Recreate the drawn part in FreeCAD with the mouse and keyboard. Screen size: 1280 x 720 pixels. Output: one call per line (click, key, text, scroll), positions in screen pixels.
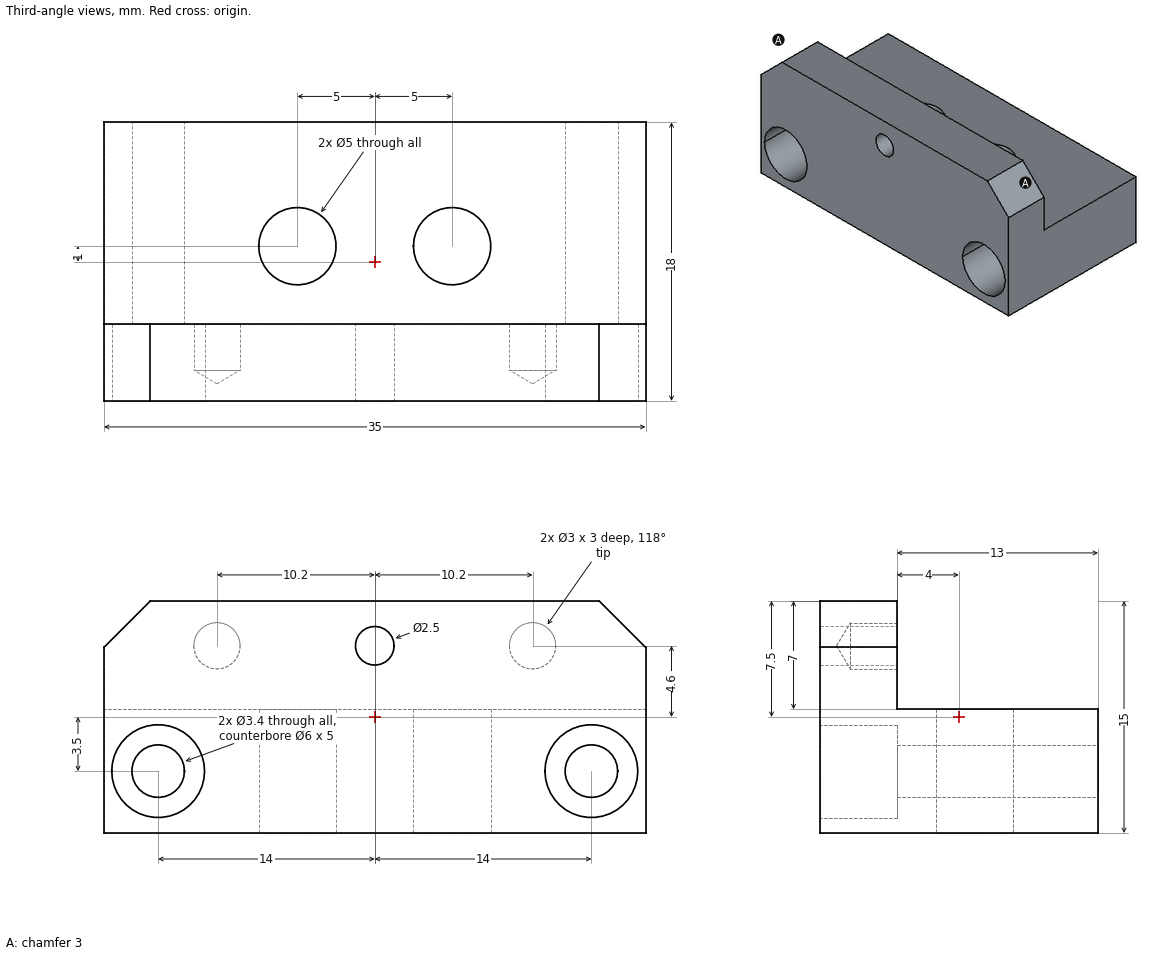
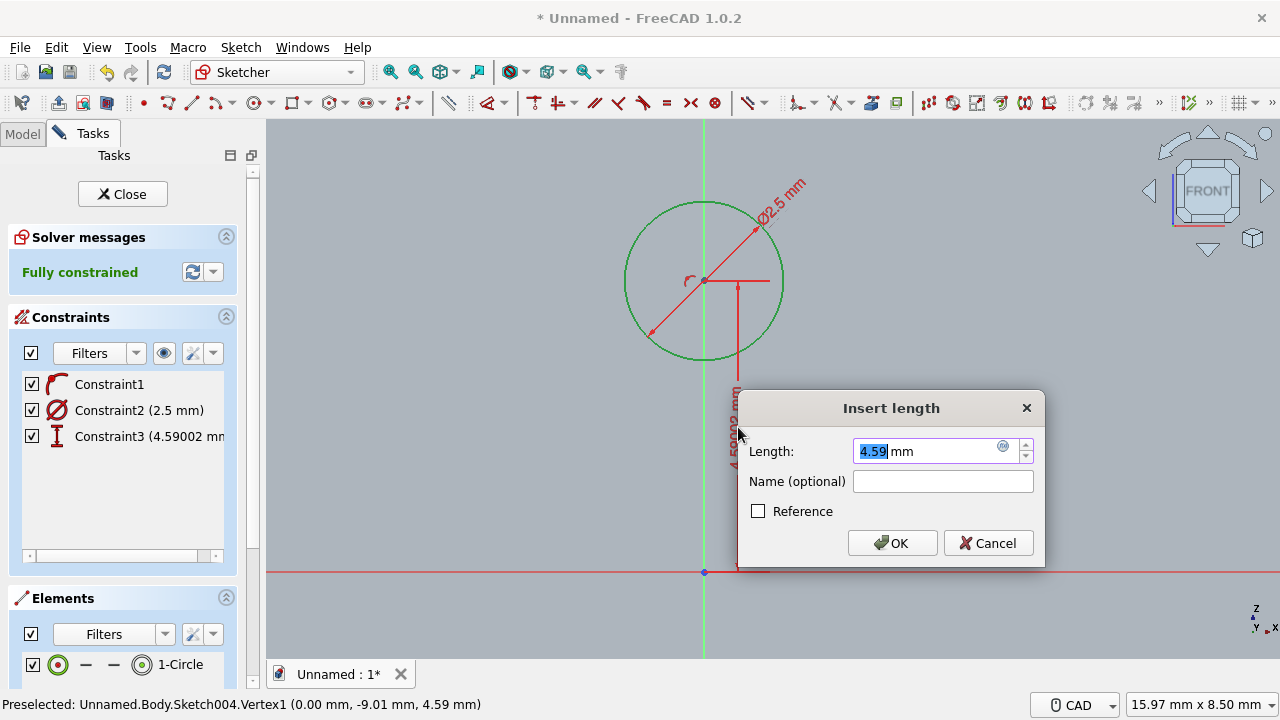
text(4.6)
key(Return)
key(Escape)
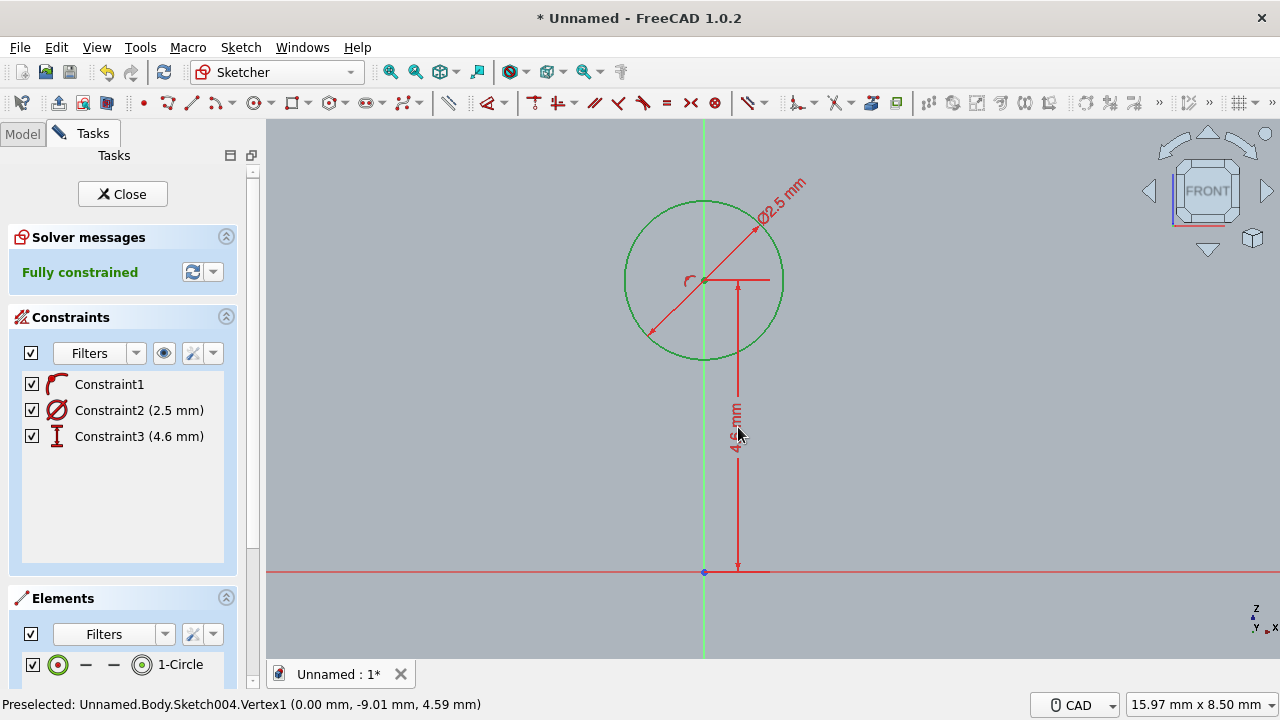
click(123, 194)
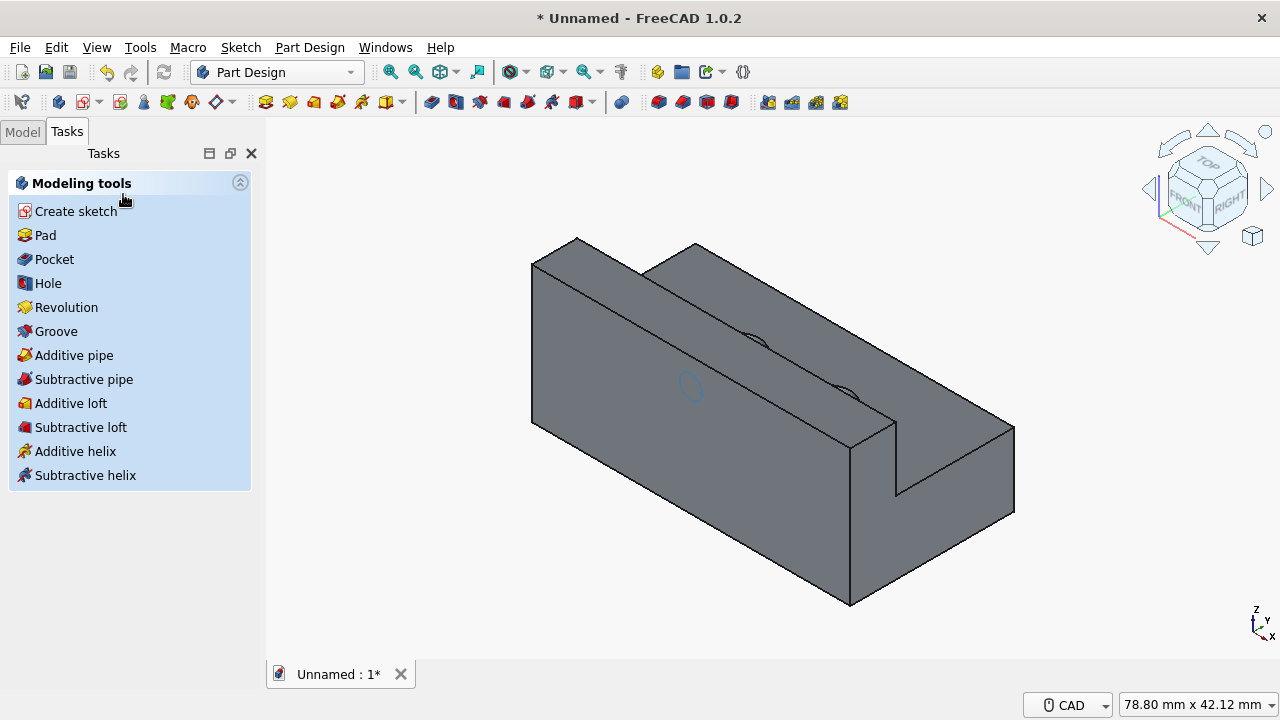
click(432, 102)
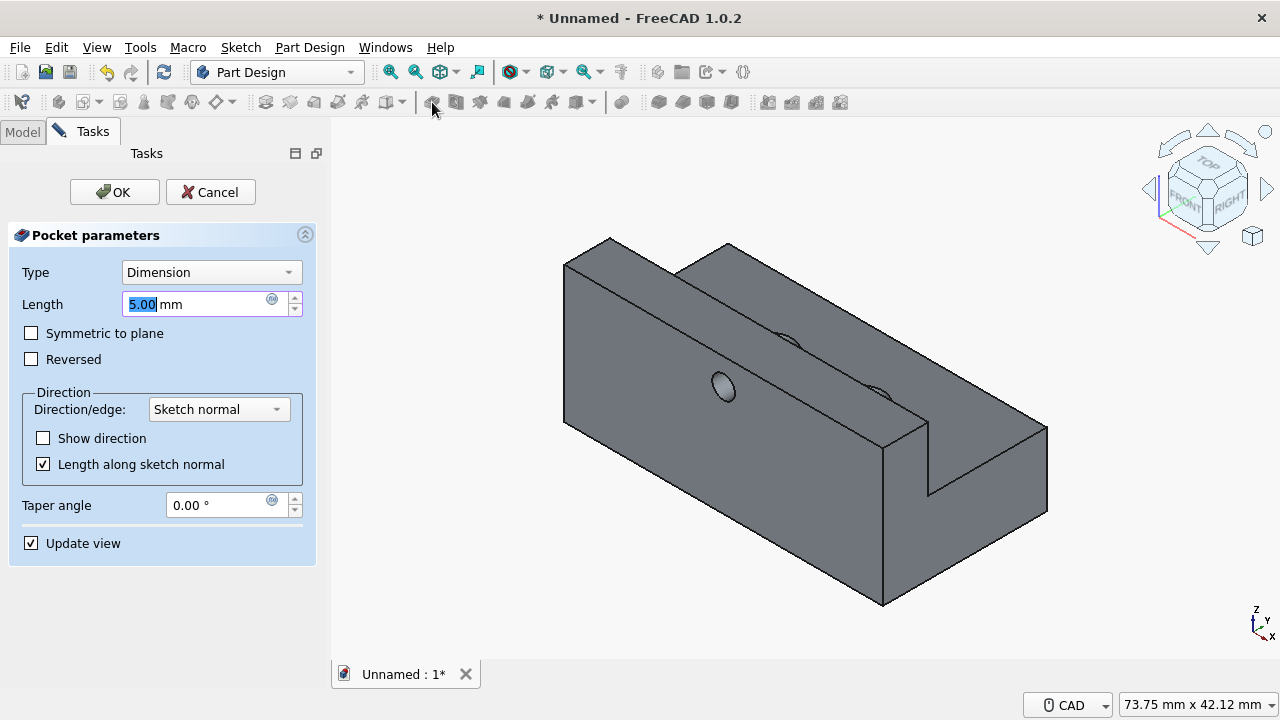
click(212, 272)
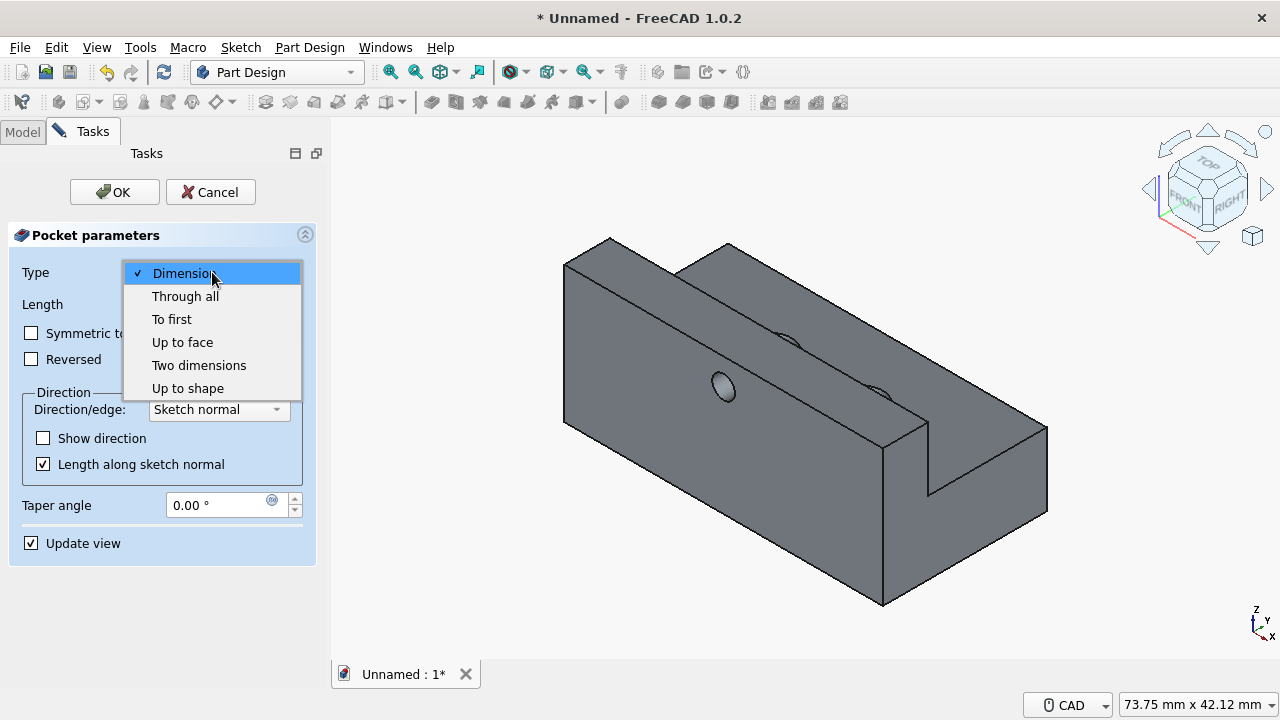
click(212, 296)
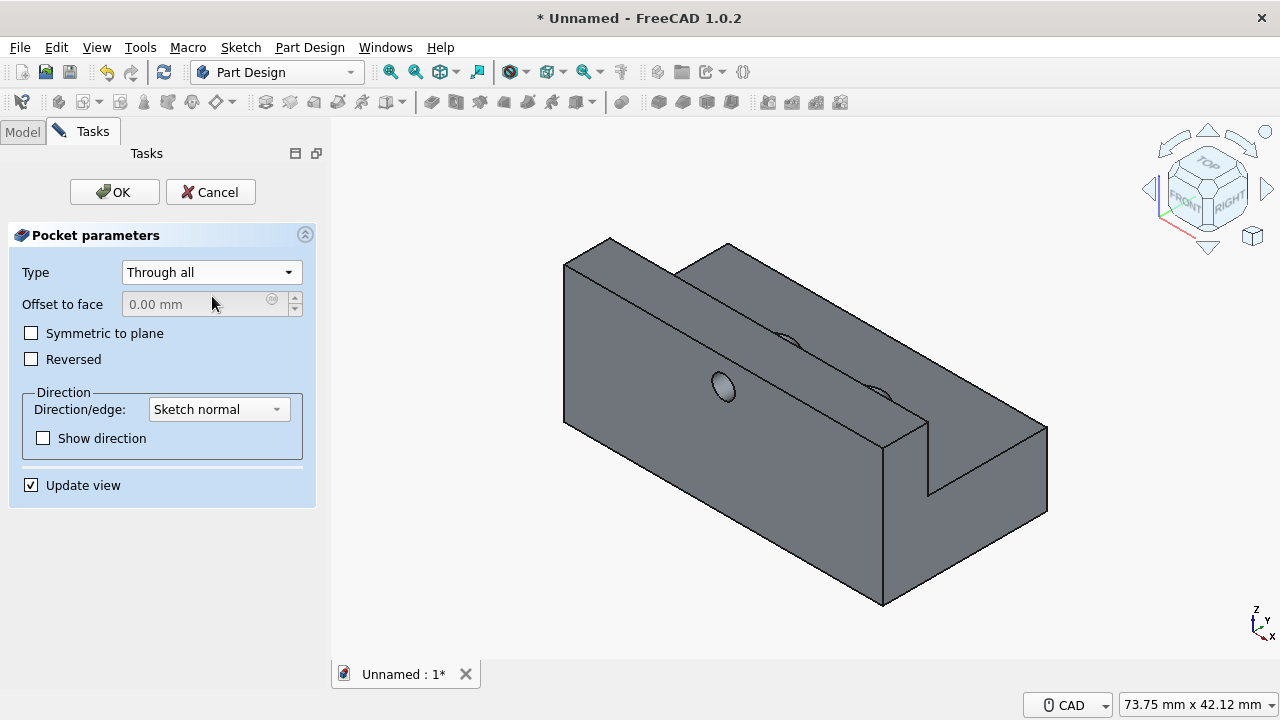
click(115, 192)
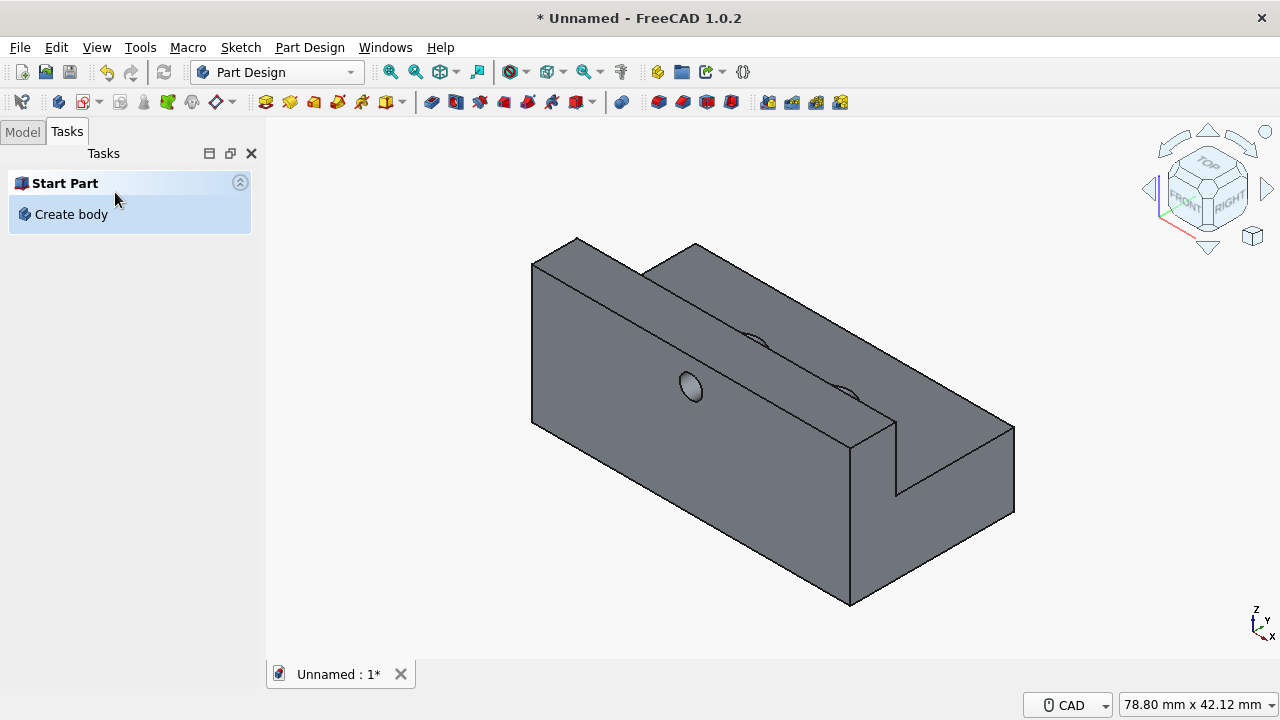
click(782, 487)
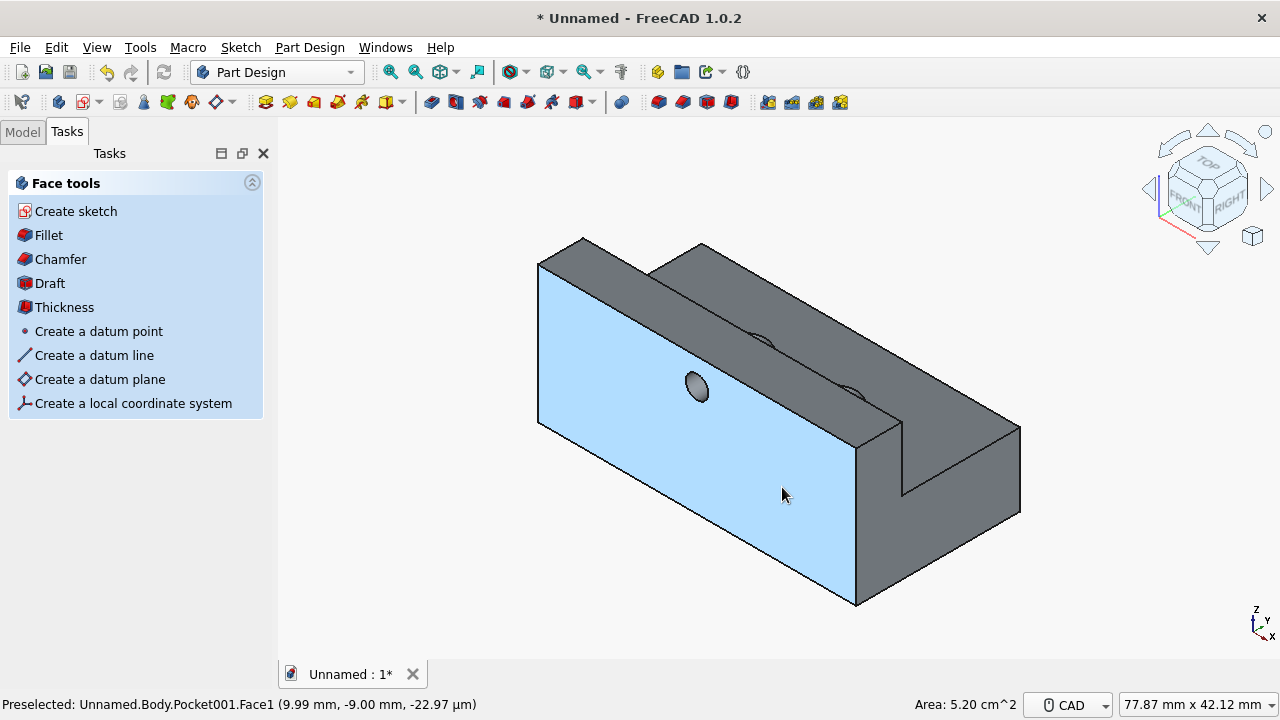
click(84, 102)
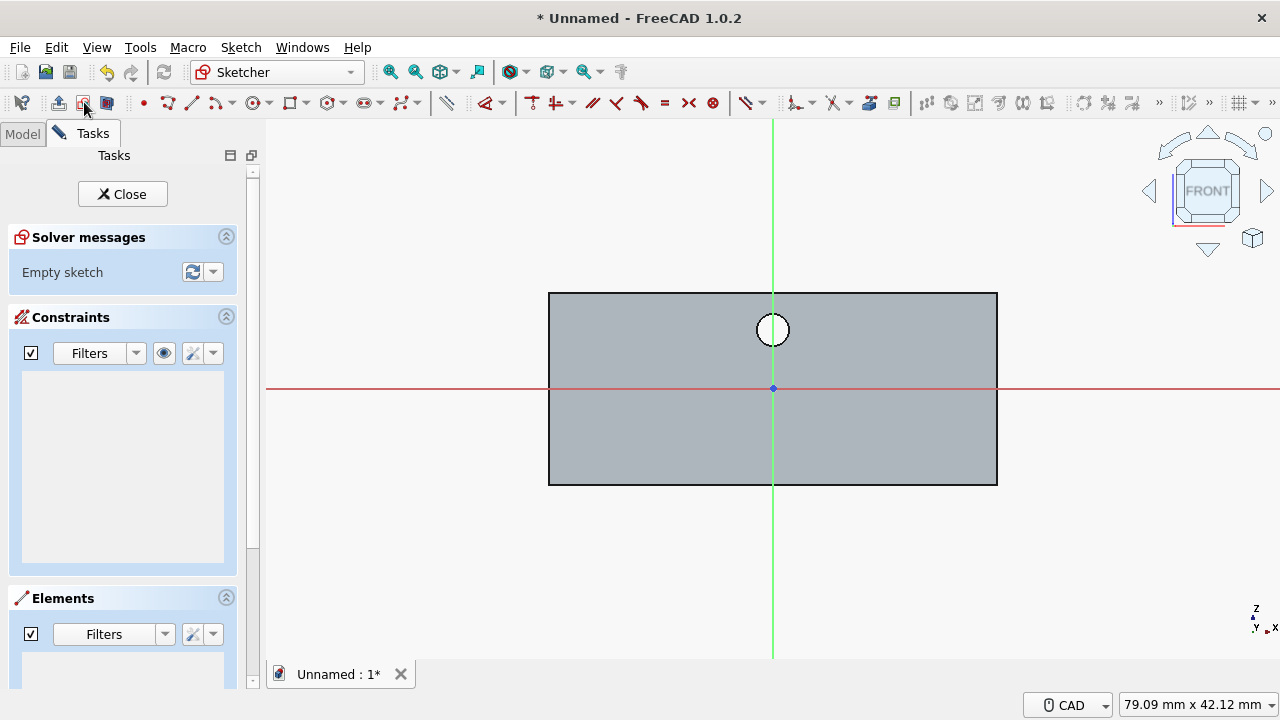
scroll(912, 490, up, 2)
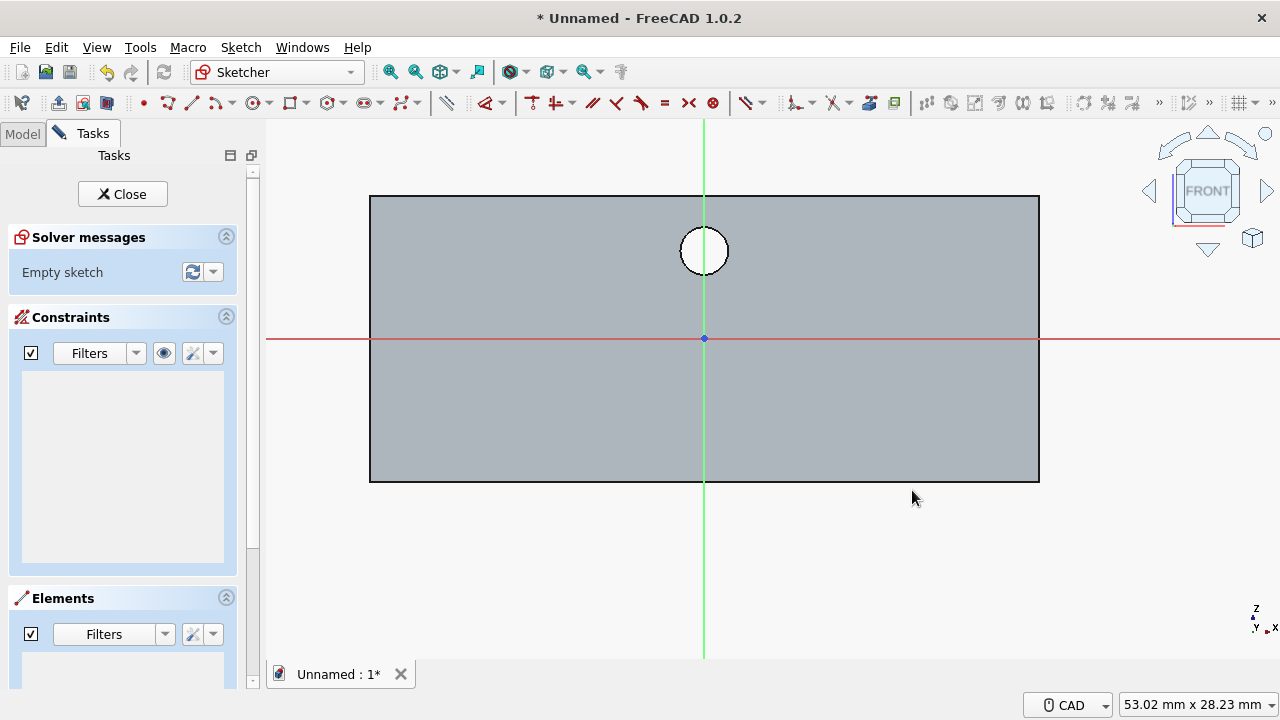
click(254, 104)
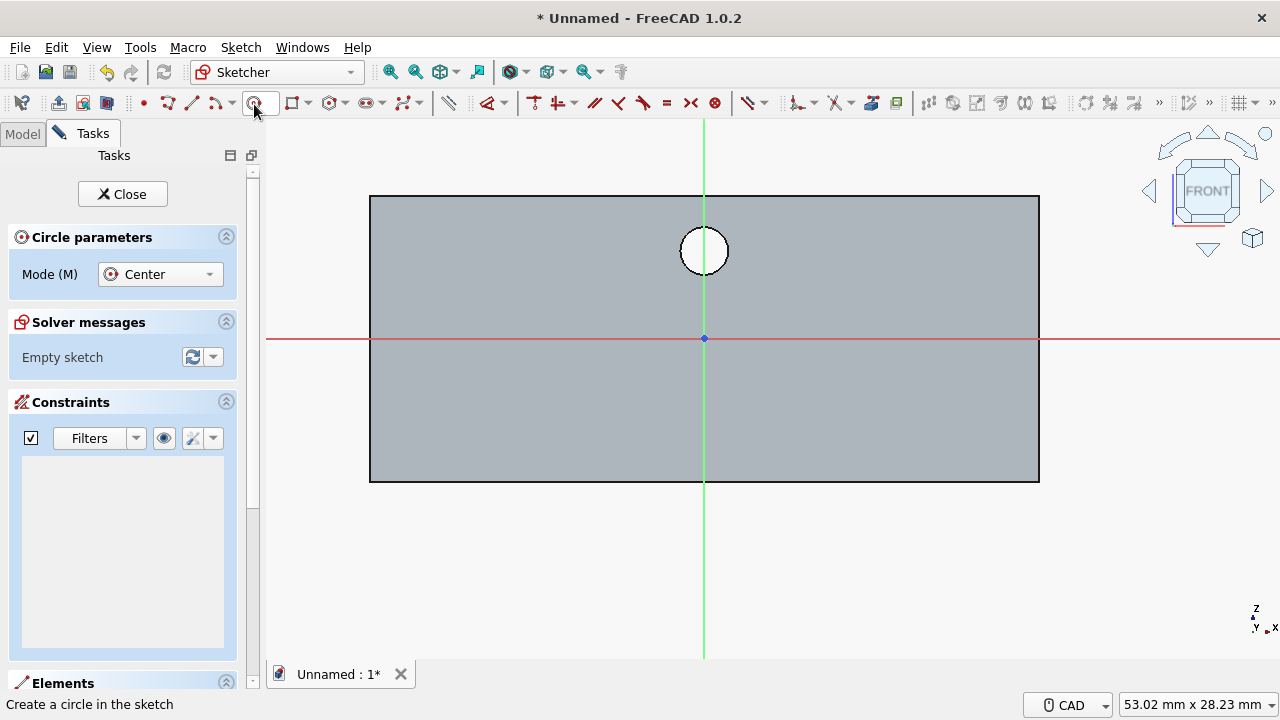
click(437, 406)
click(460, 383)